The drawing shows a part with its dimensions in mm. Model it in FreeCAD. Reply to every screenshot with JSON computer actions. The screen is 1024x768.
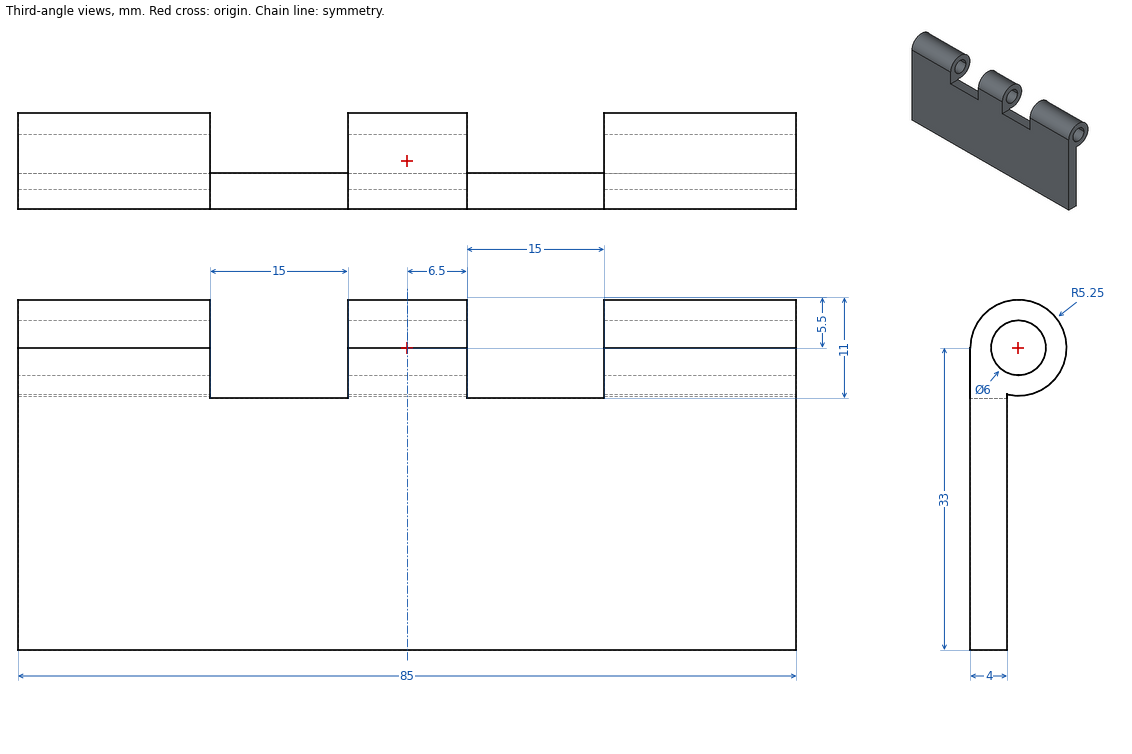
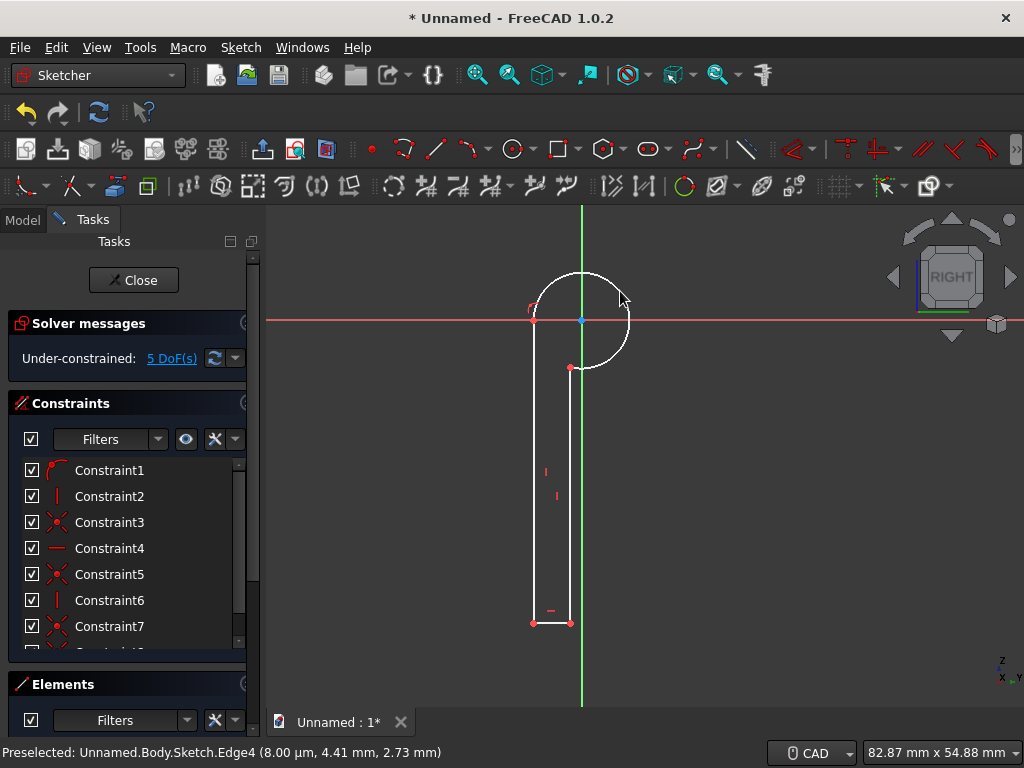
{"action": "left_click", "coordinate": [534, 411]}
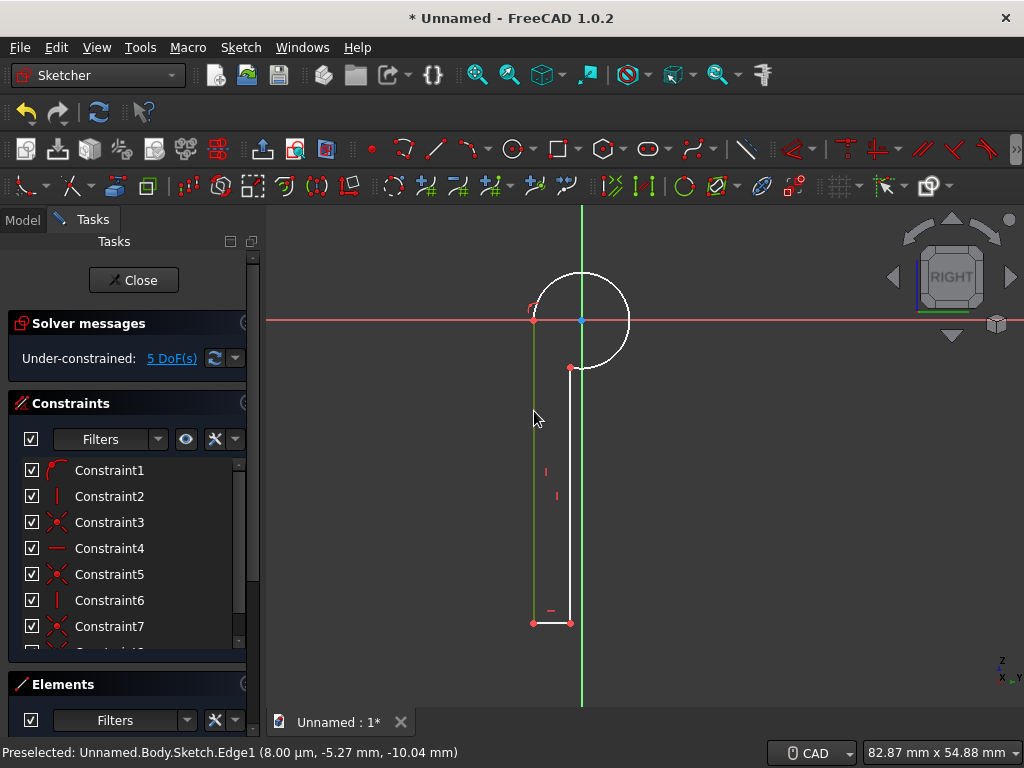
{"action": "left_click", "coordinate": [627, 336]}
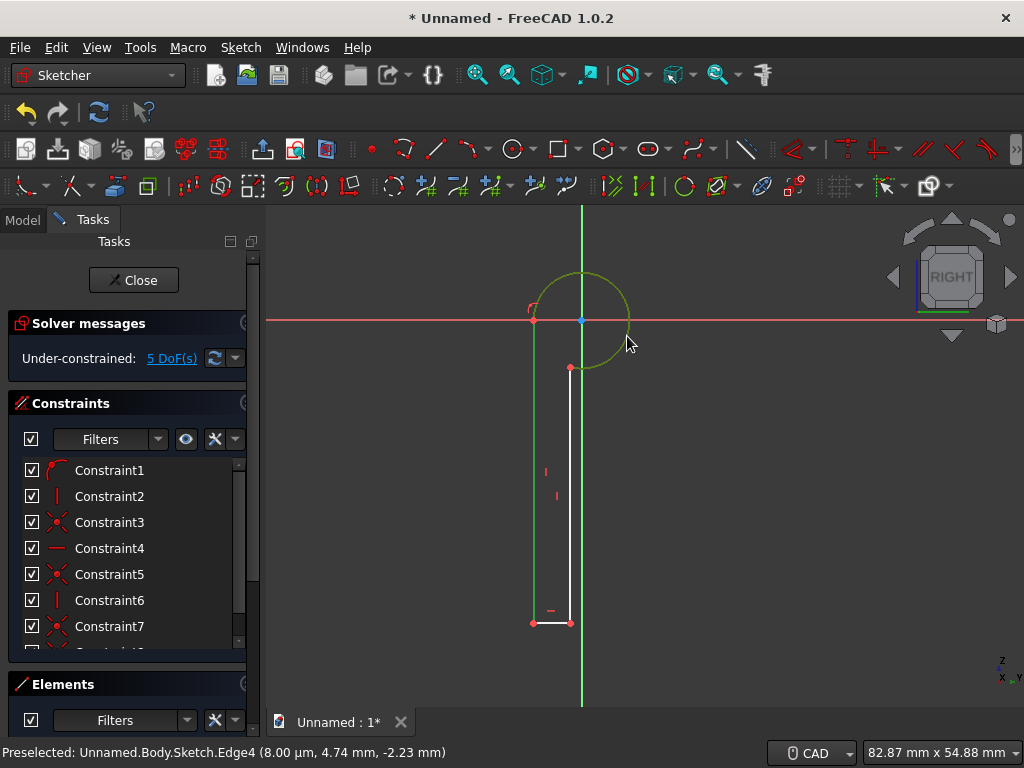
{"action": "left_click", "coordinate": [988, 150]}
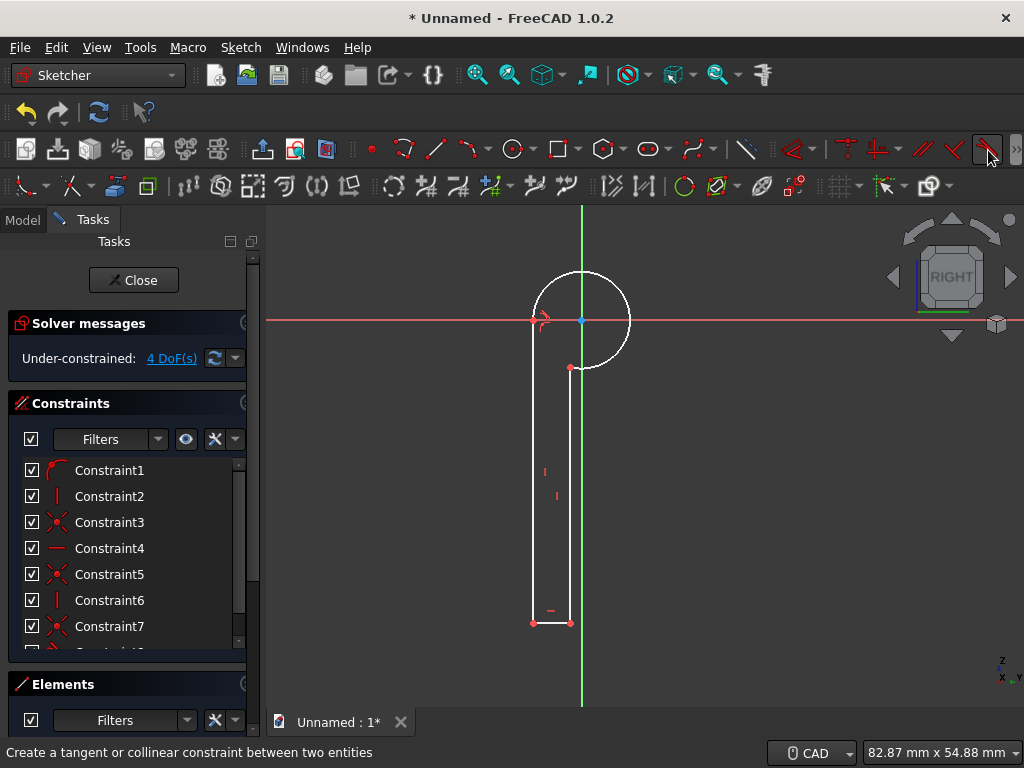
{"action": "left_click", "coordinate": [582, 320]}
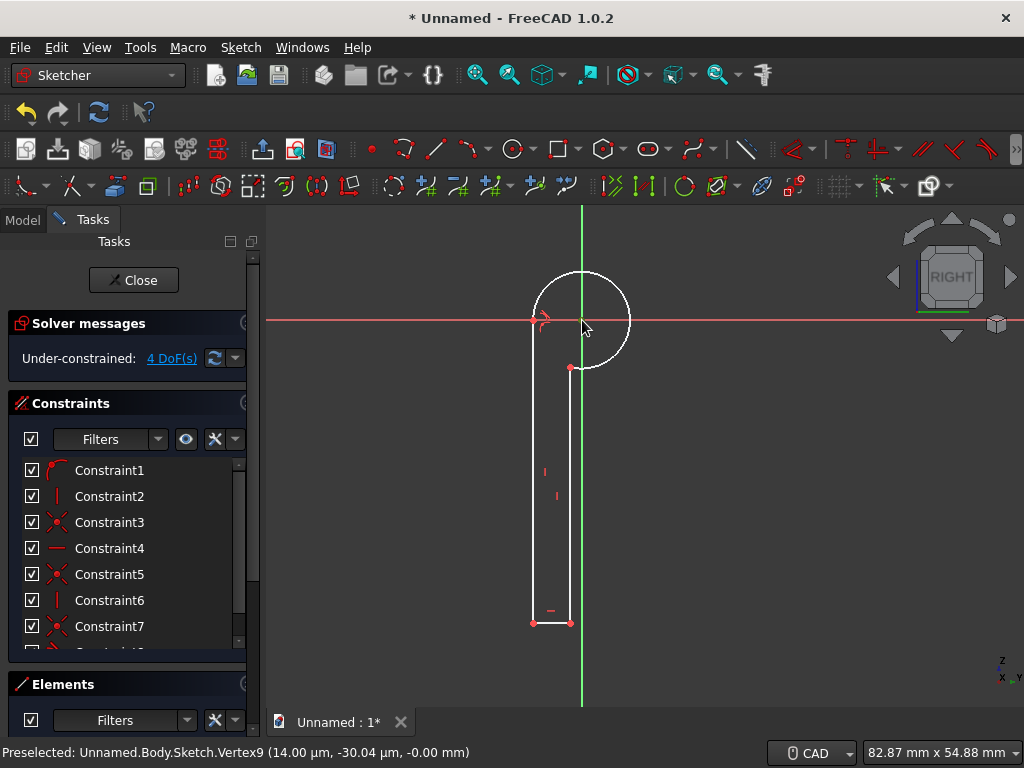
{"action": "left_click", "coordinate": [582, 647]}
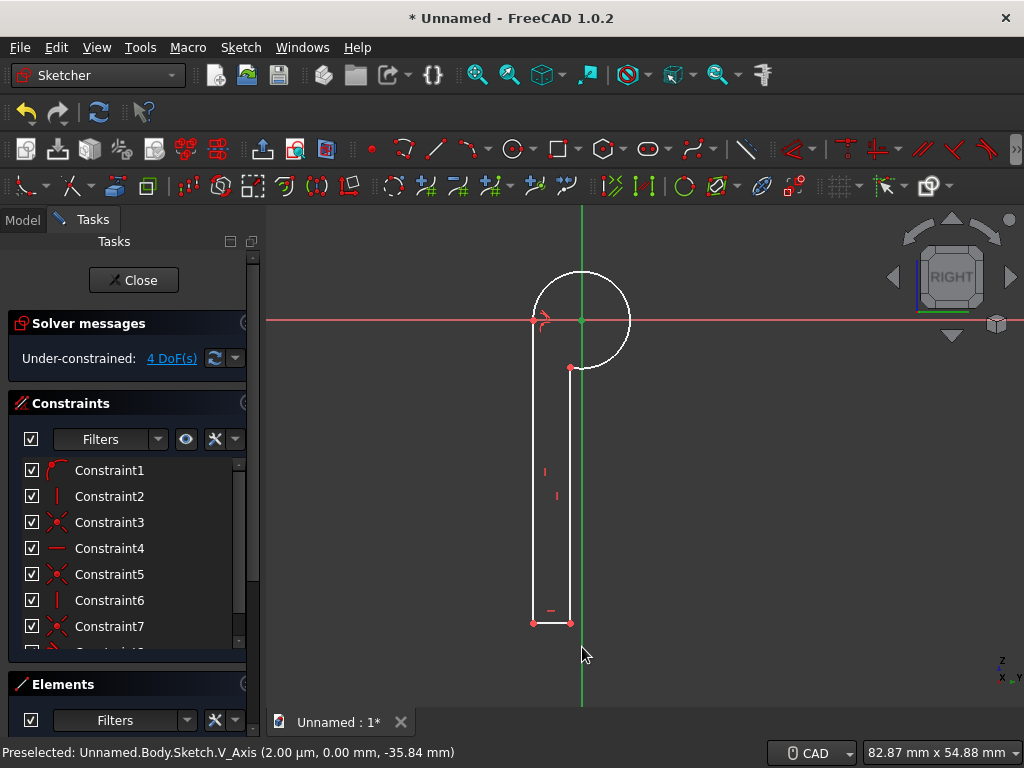
{"action": "left_click", "coordinate": [846, 150]}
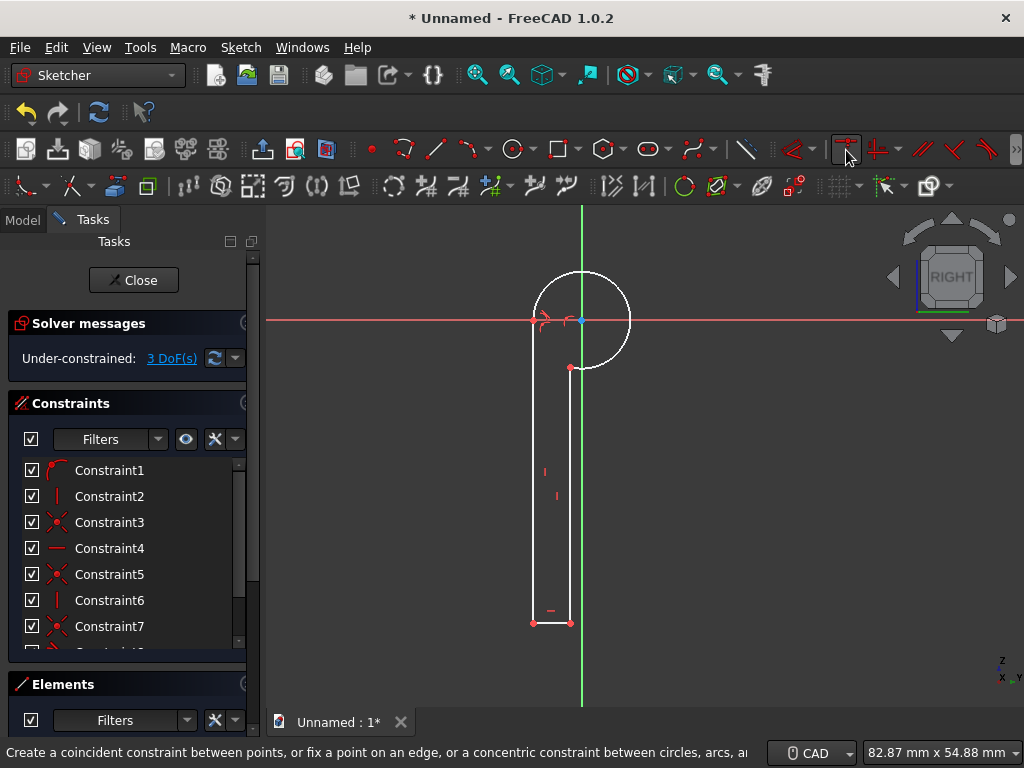
{"action": "left_click", "coordinate": [792, 150]}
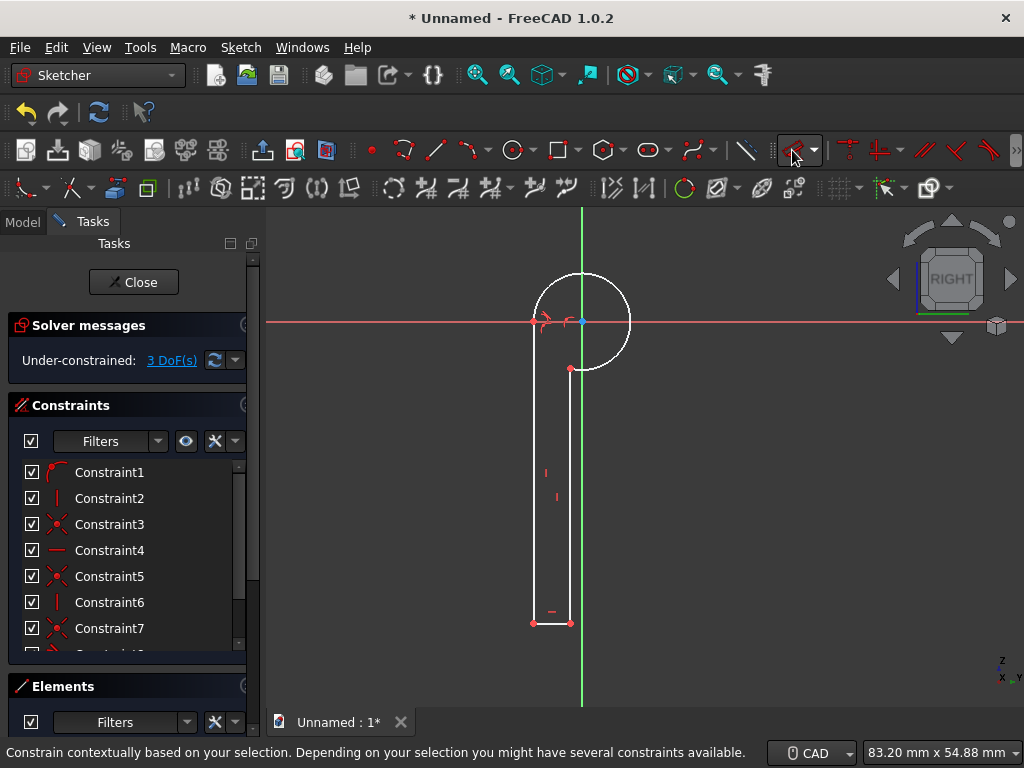
{"action": "left_click", "coordinate": [628, 337]}
{"action": "left_click", "coordinate": [658, 347]}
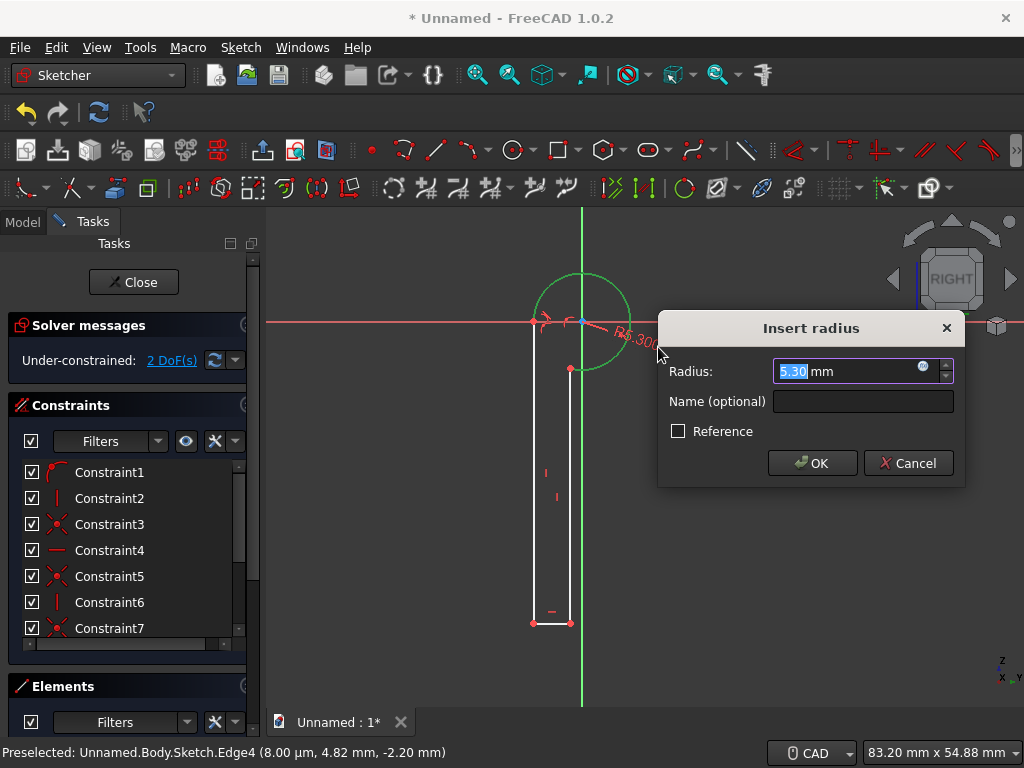
{"action": "type", "text": "5.25"}
{"action": "key", "text": "Return"}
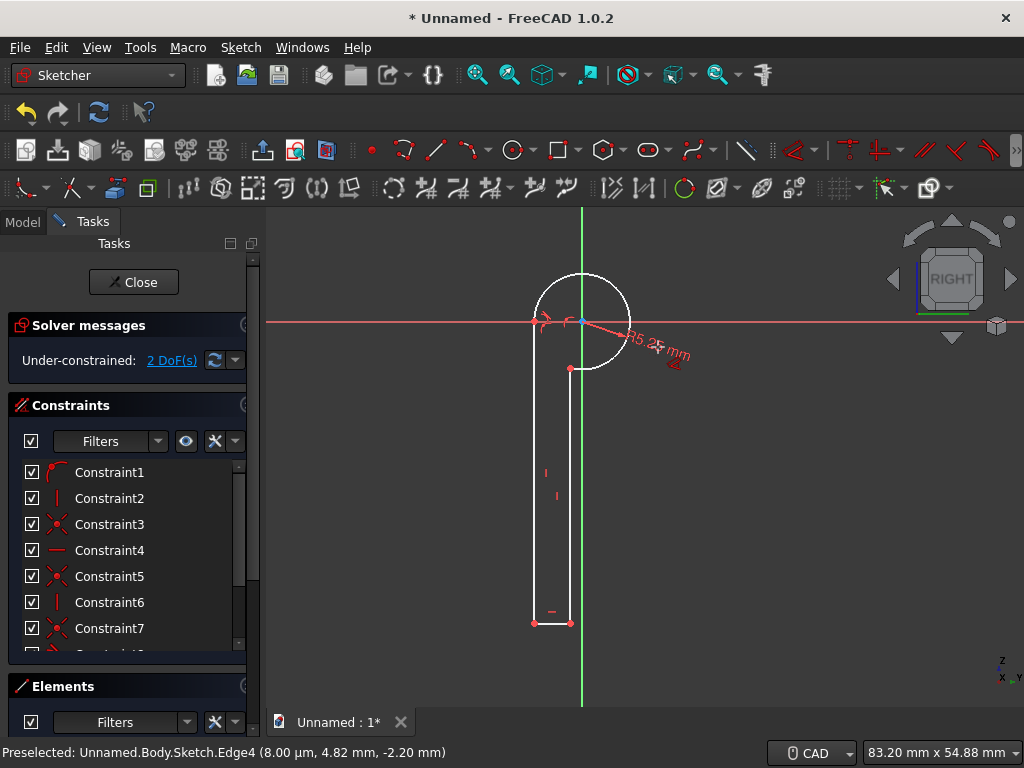
{"action": "scroll", "coordinate": [545, 624], "scroll_direction": "up", "scroll_amount": 2}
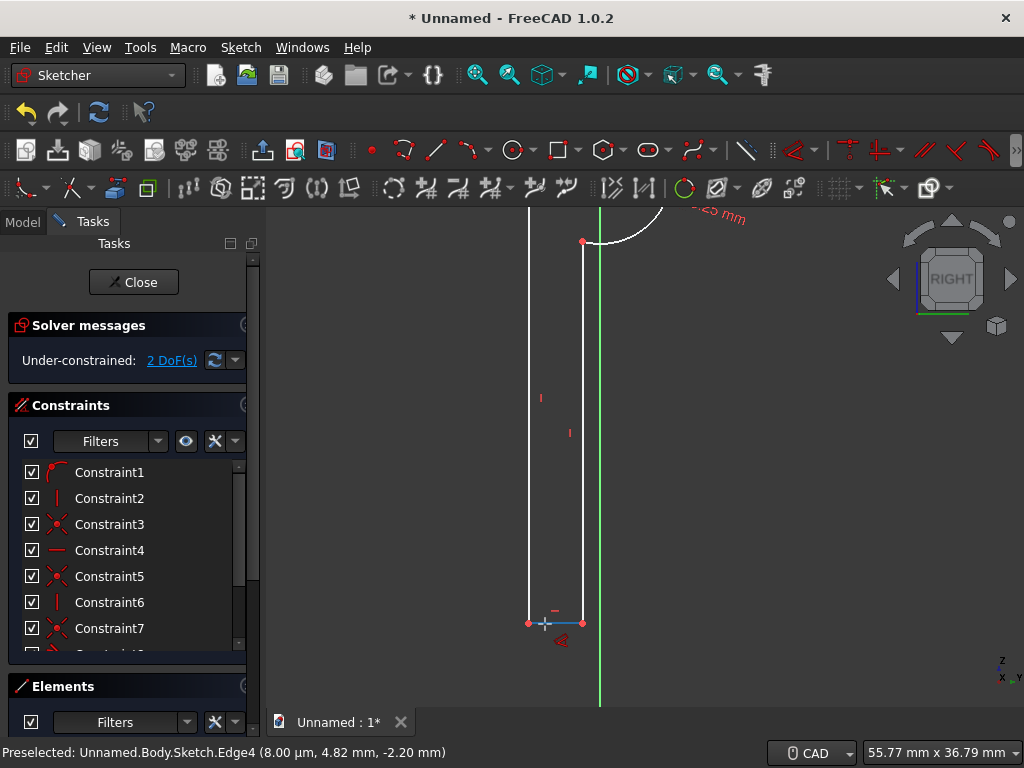
{"action": "left_click", "coordinate": [545, 623]}
{"action": "left_click", "coordinate": [556, 657]}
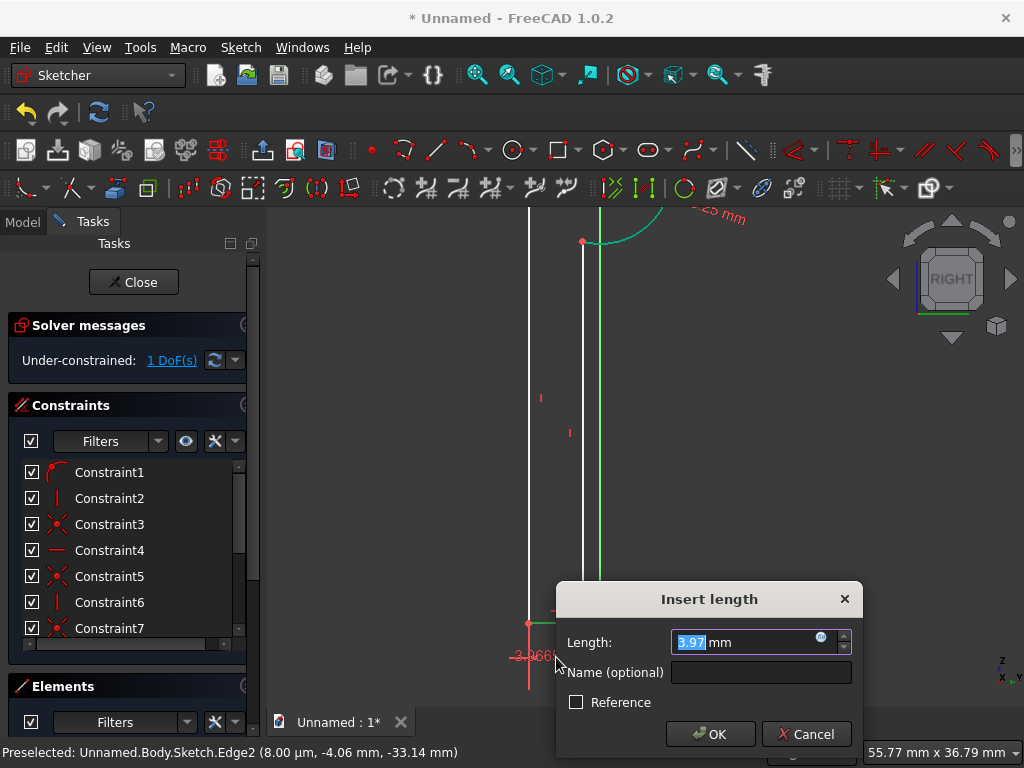
{"action": "type", "text": "4"}
{"action": "key", "text": "Return"}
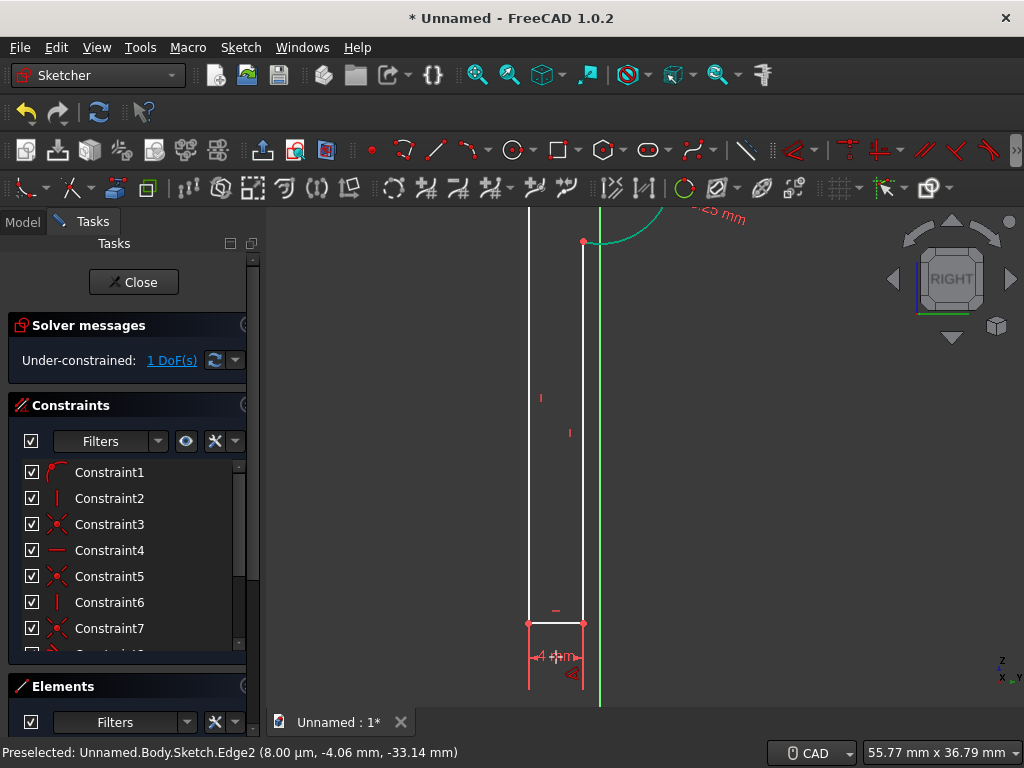
{"action": "left_click", "coordinate": [529, 308]}
{"action": "left_click", "coordinate": [495, 429]}